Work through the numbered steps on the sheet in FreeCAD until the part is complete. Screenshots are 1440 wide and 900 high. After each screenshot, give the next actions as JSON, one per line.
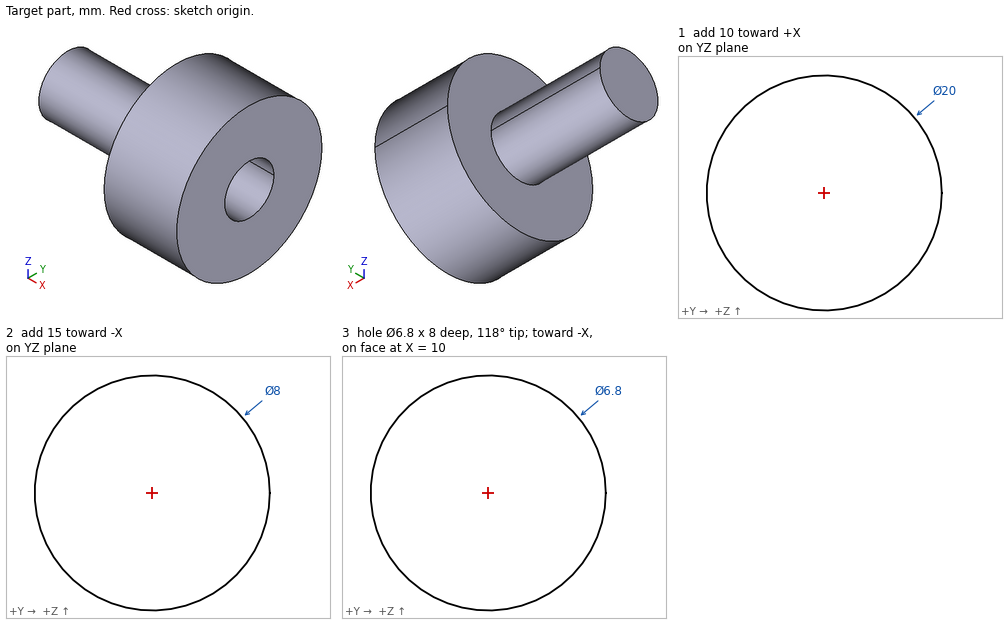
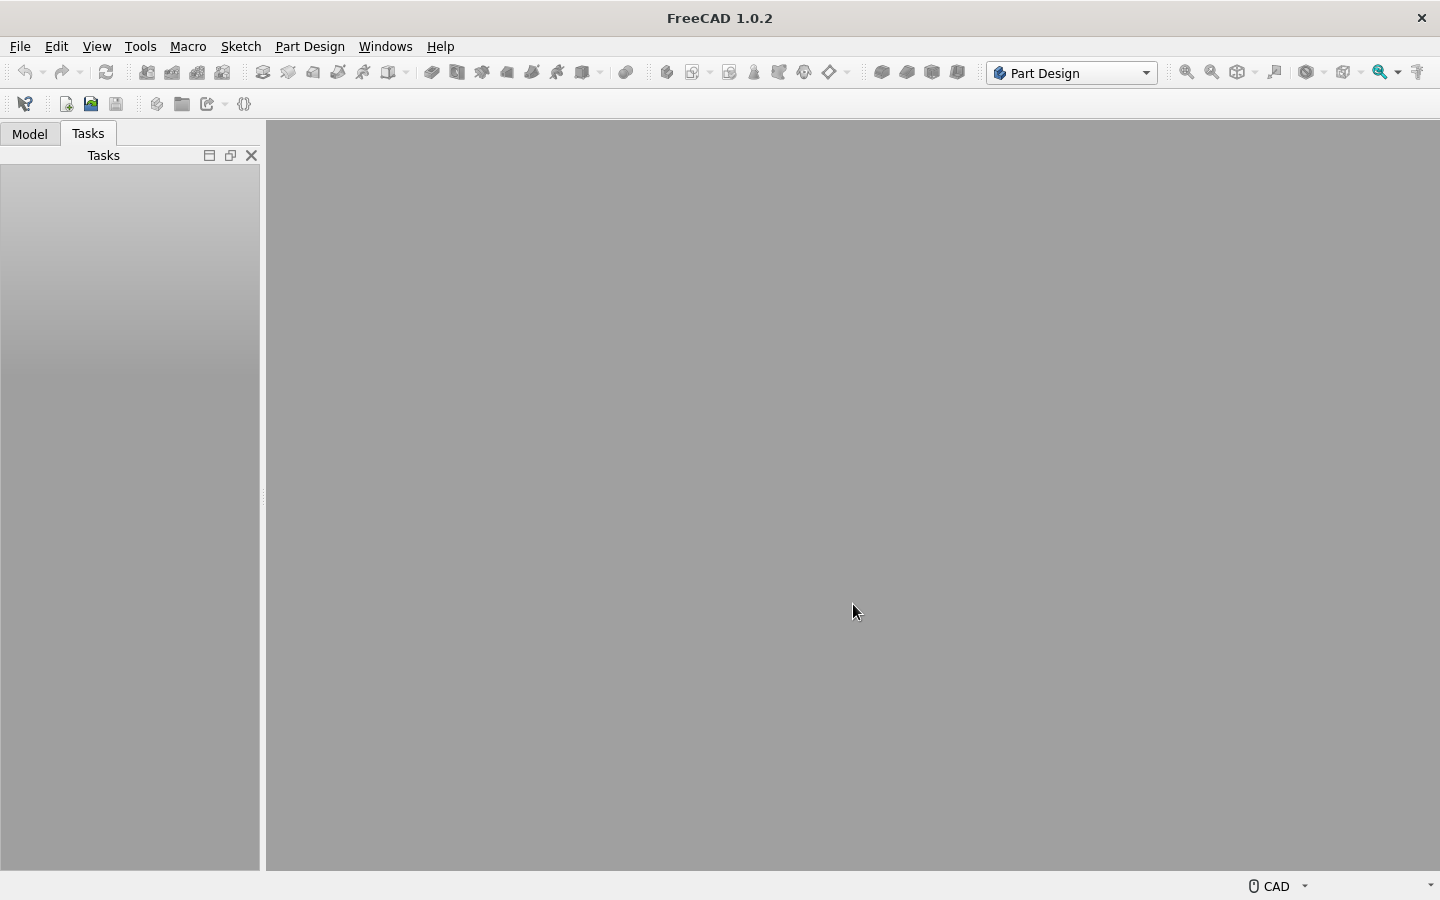
{"action": "left_click", "coordinate": [66, 104]}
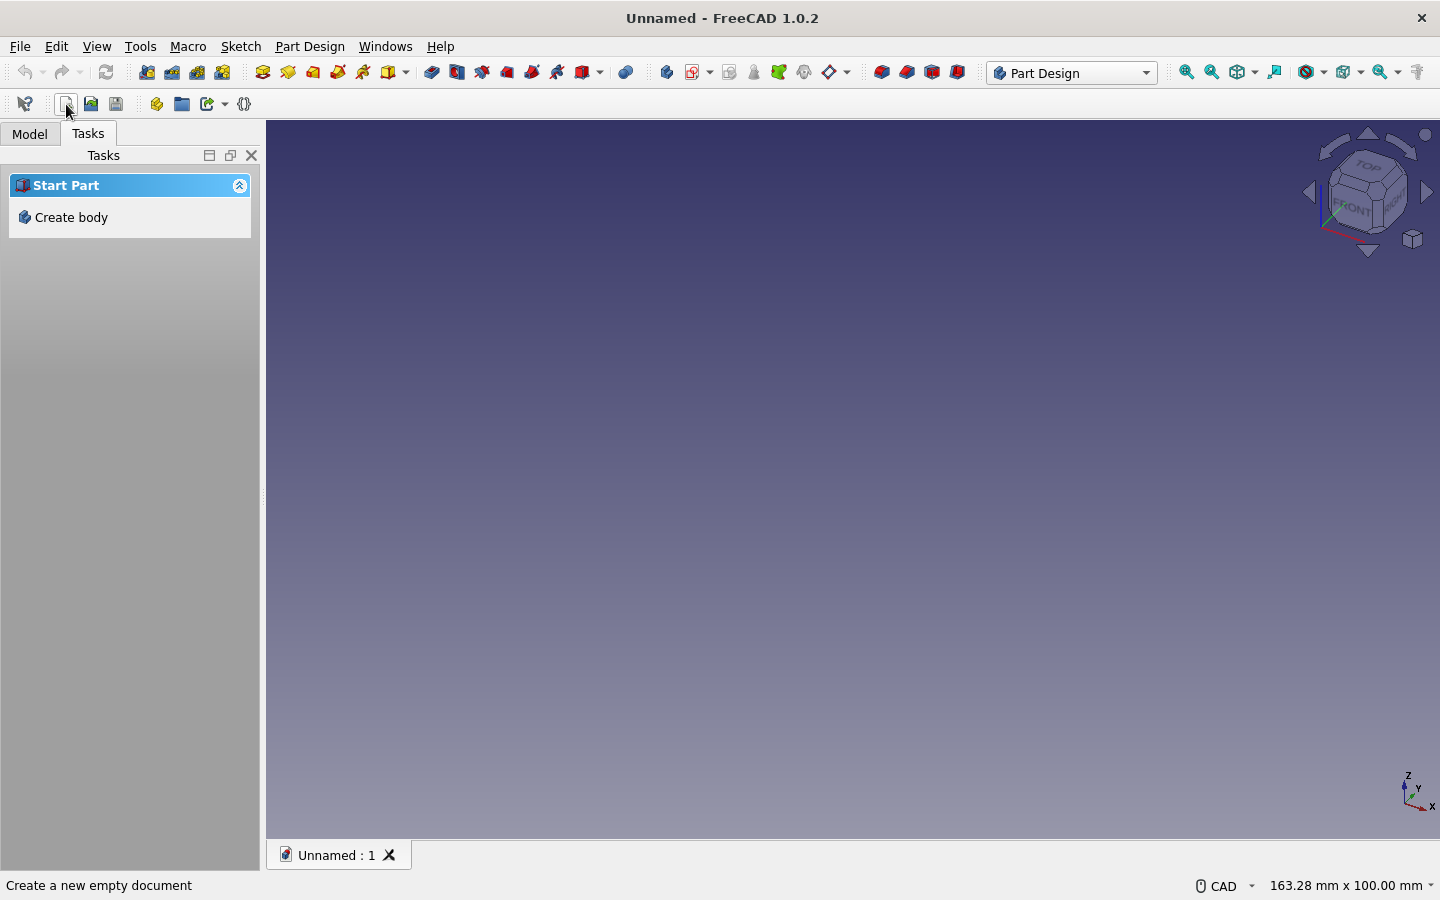
{"action": "left_click", "coordinate": [692, 72]}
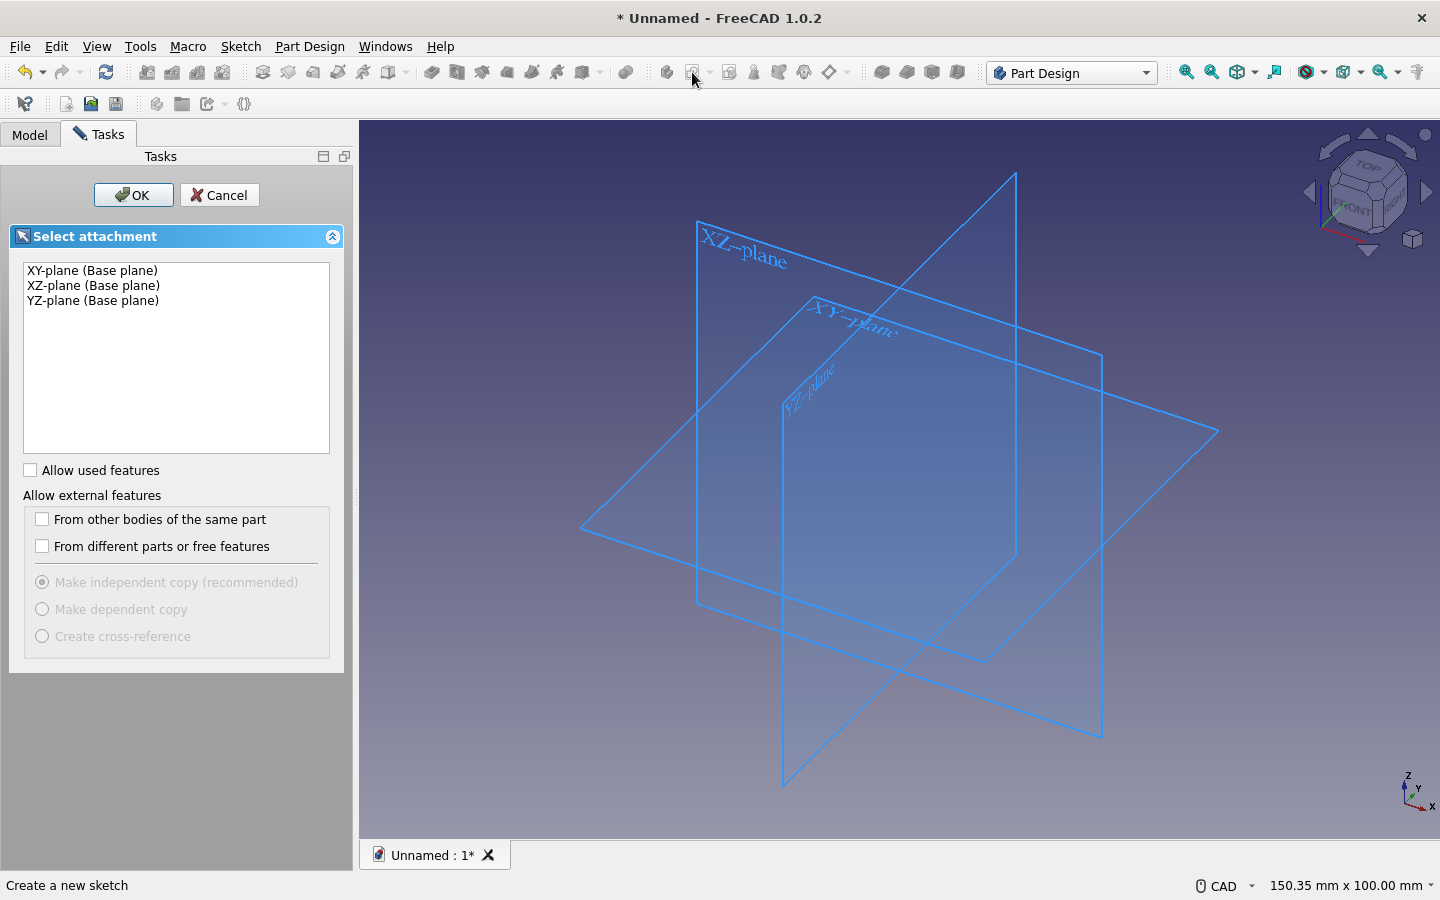
{"action": "left_click", "coordinate": [84, 300]}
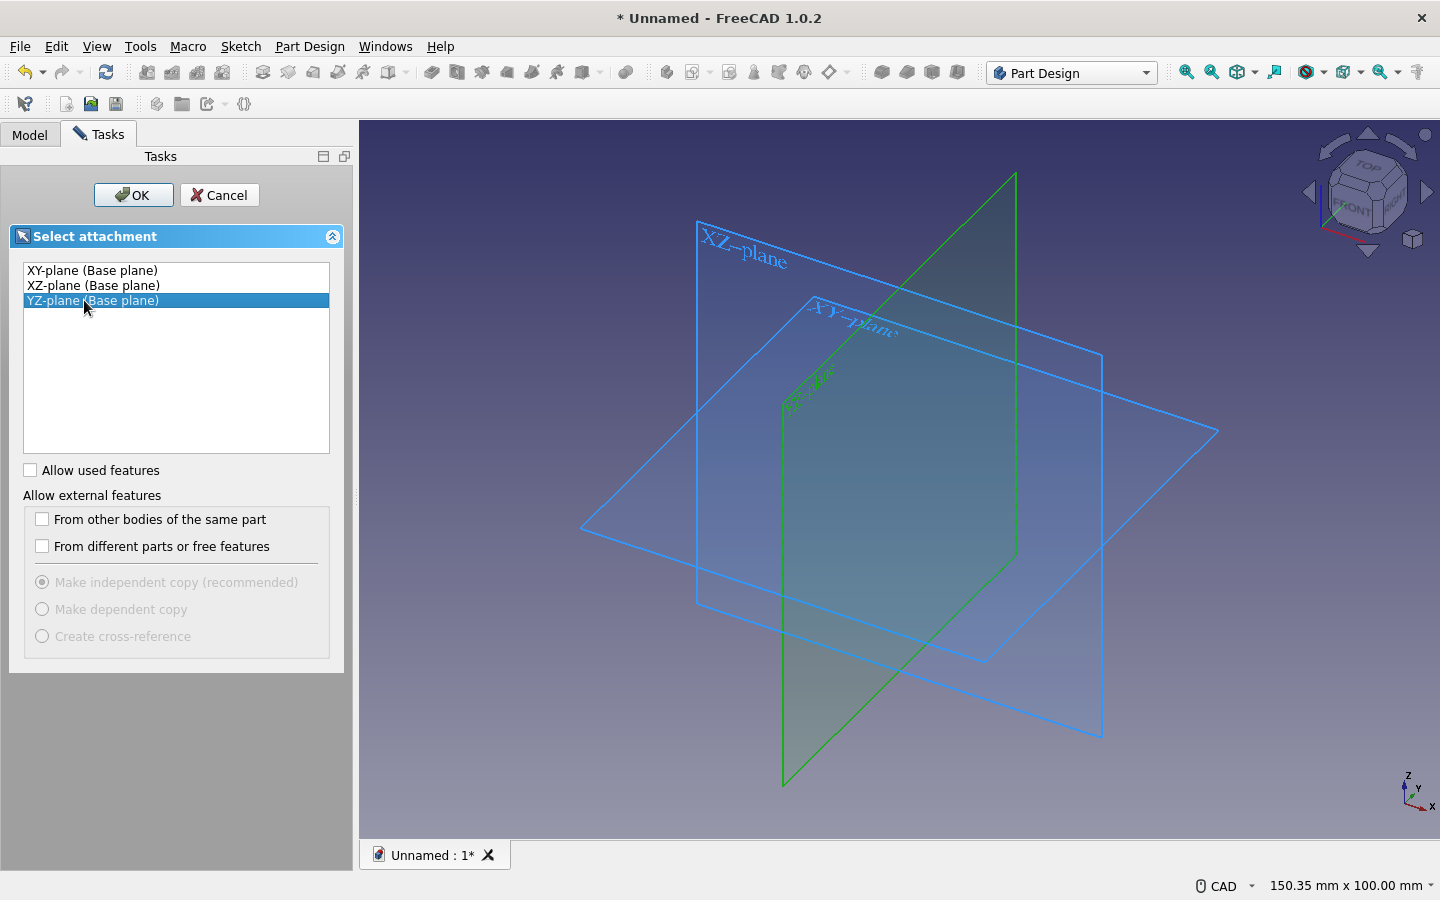
{"action": "left_click", "coordinate": [134, 195]}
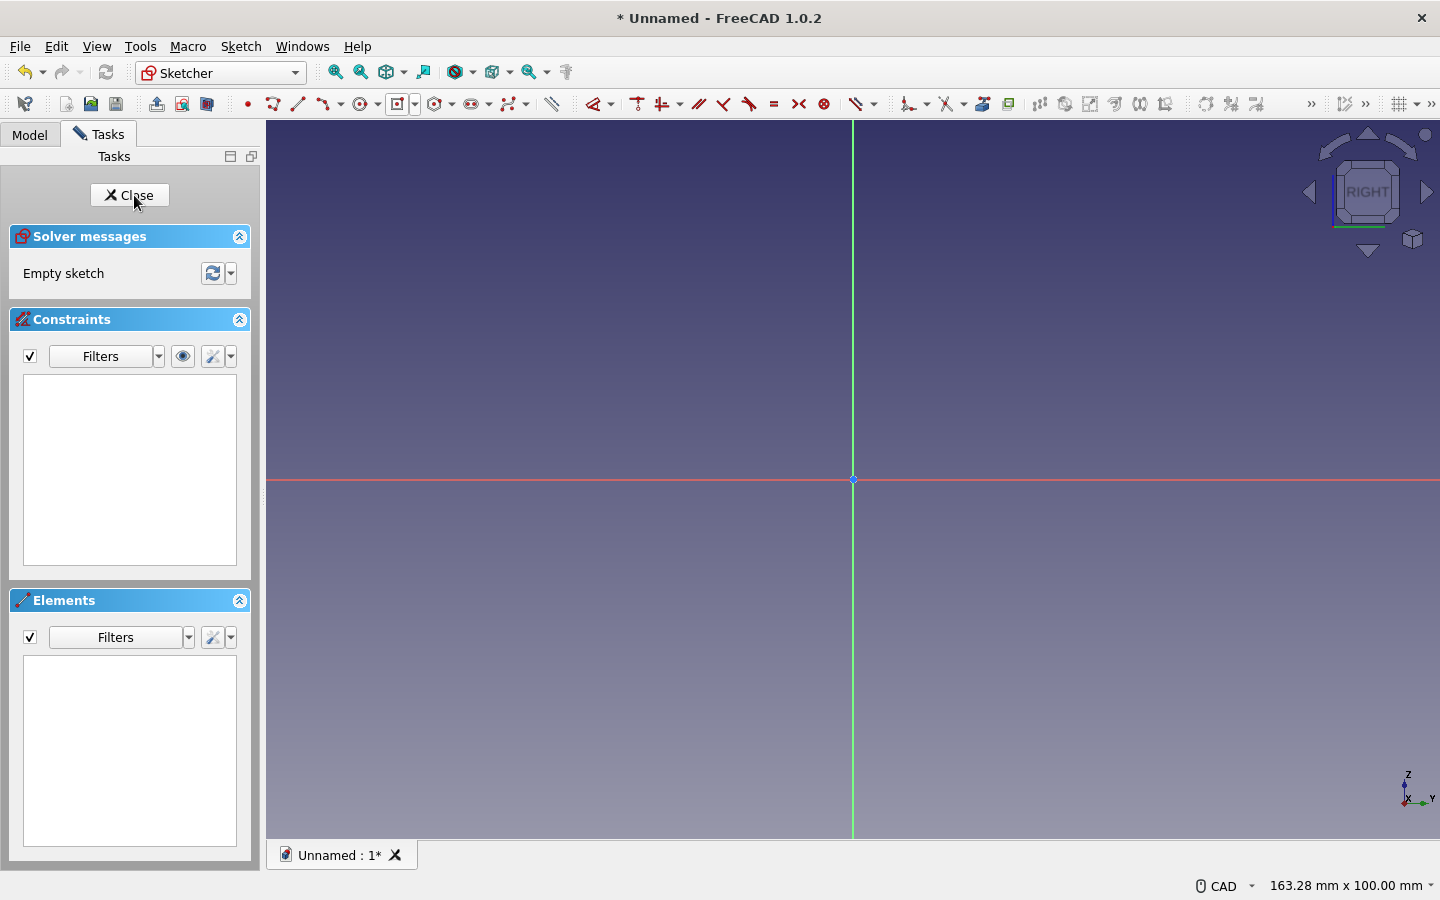
{"action": "scroll", "coordinate": [883, 480], "scroll_direction": "up", "scroll_amount": 6}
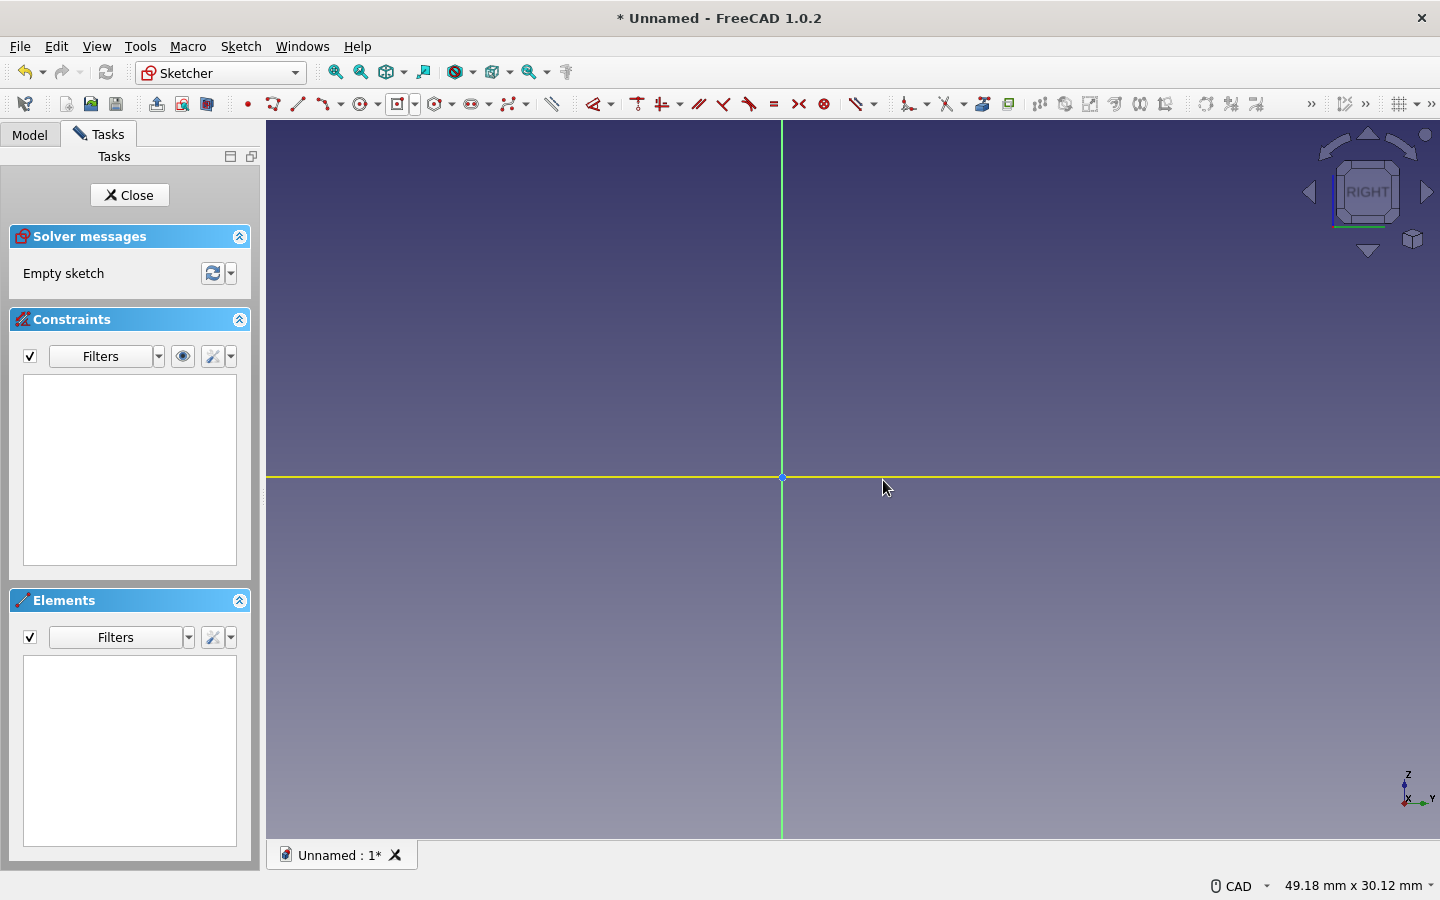
{"action": "left_click", "coordinate": [360, 104]}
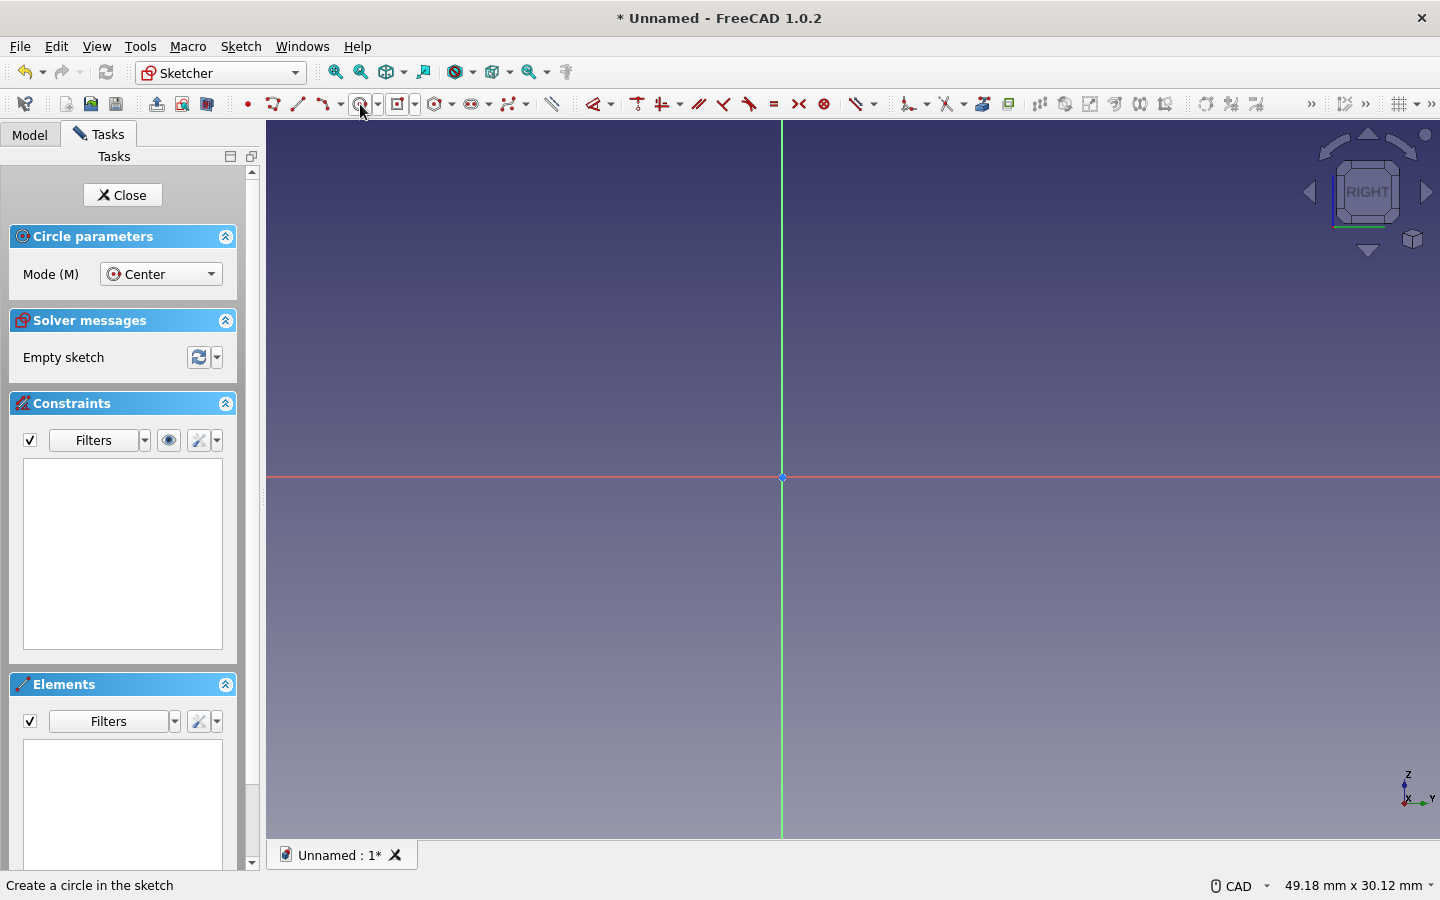
{"action": "left_click", "coordinate": [782, 477]}
{"action": "left_click", "coordinate": [951, 308]}
{"action": "key", "text": "Escape"}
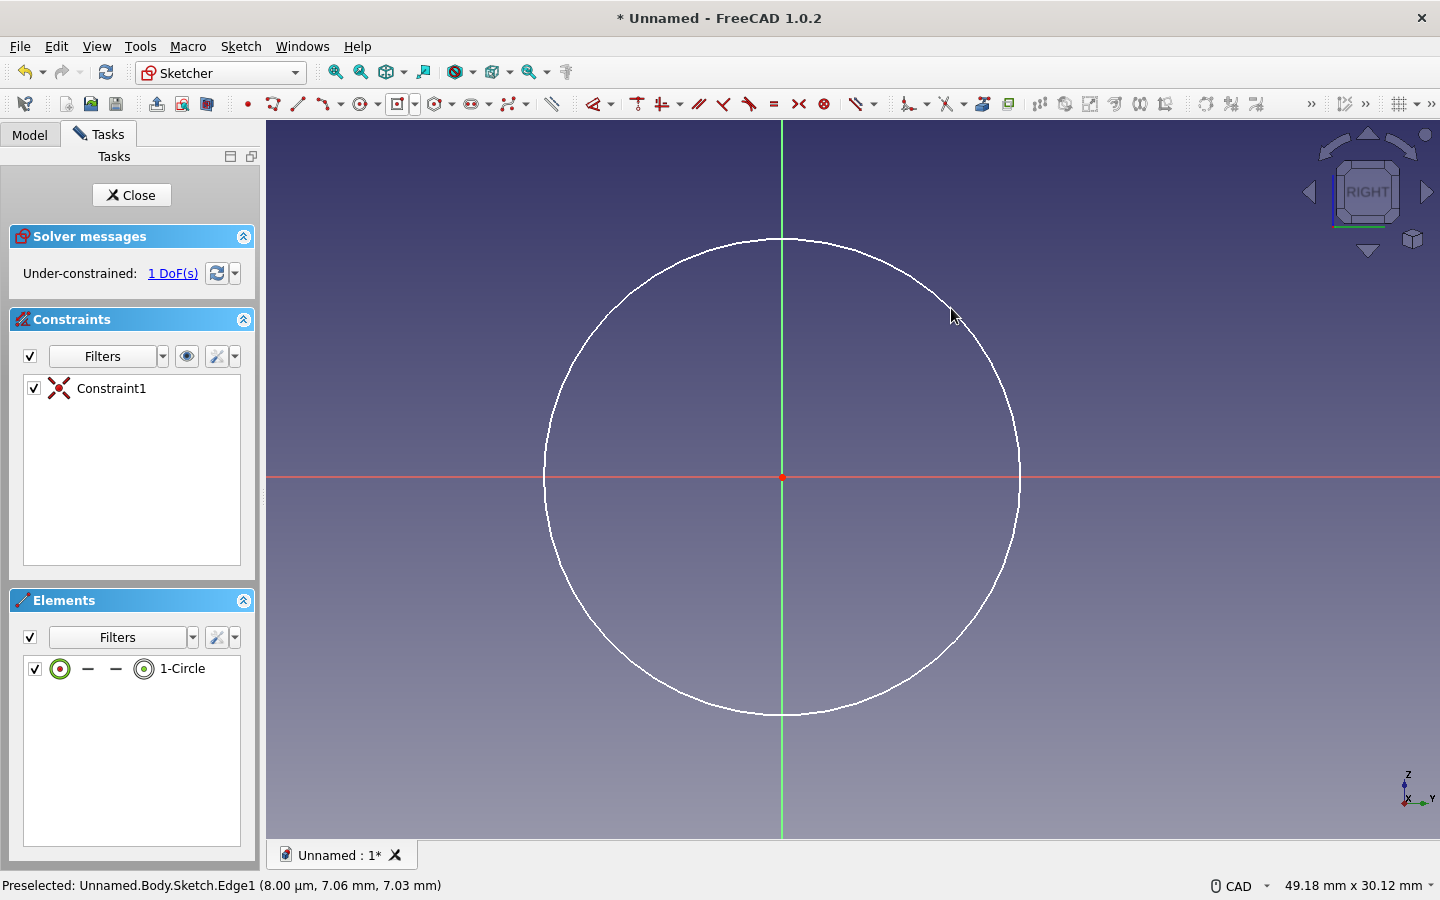
{"action": "left_click", "coordinate": [592, 104]}